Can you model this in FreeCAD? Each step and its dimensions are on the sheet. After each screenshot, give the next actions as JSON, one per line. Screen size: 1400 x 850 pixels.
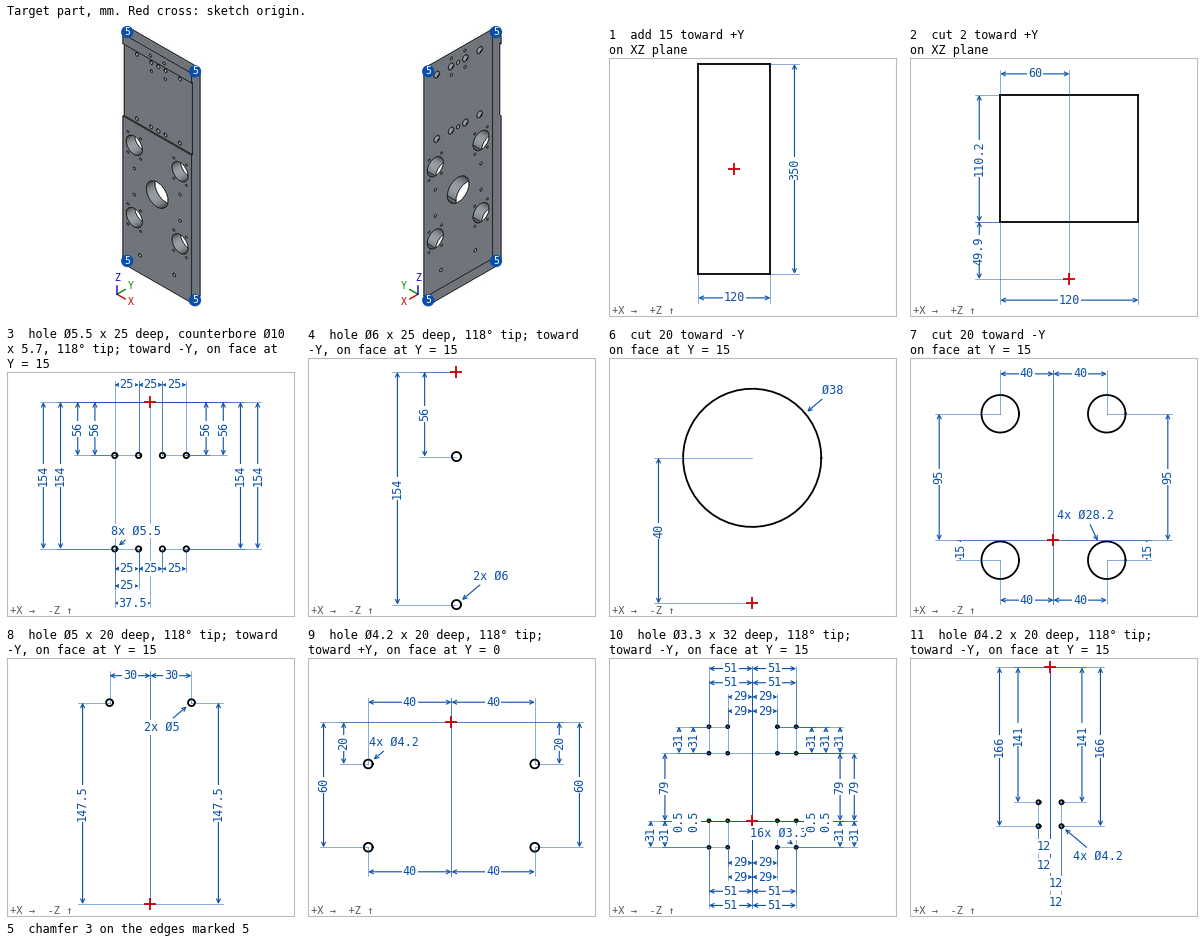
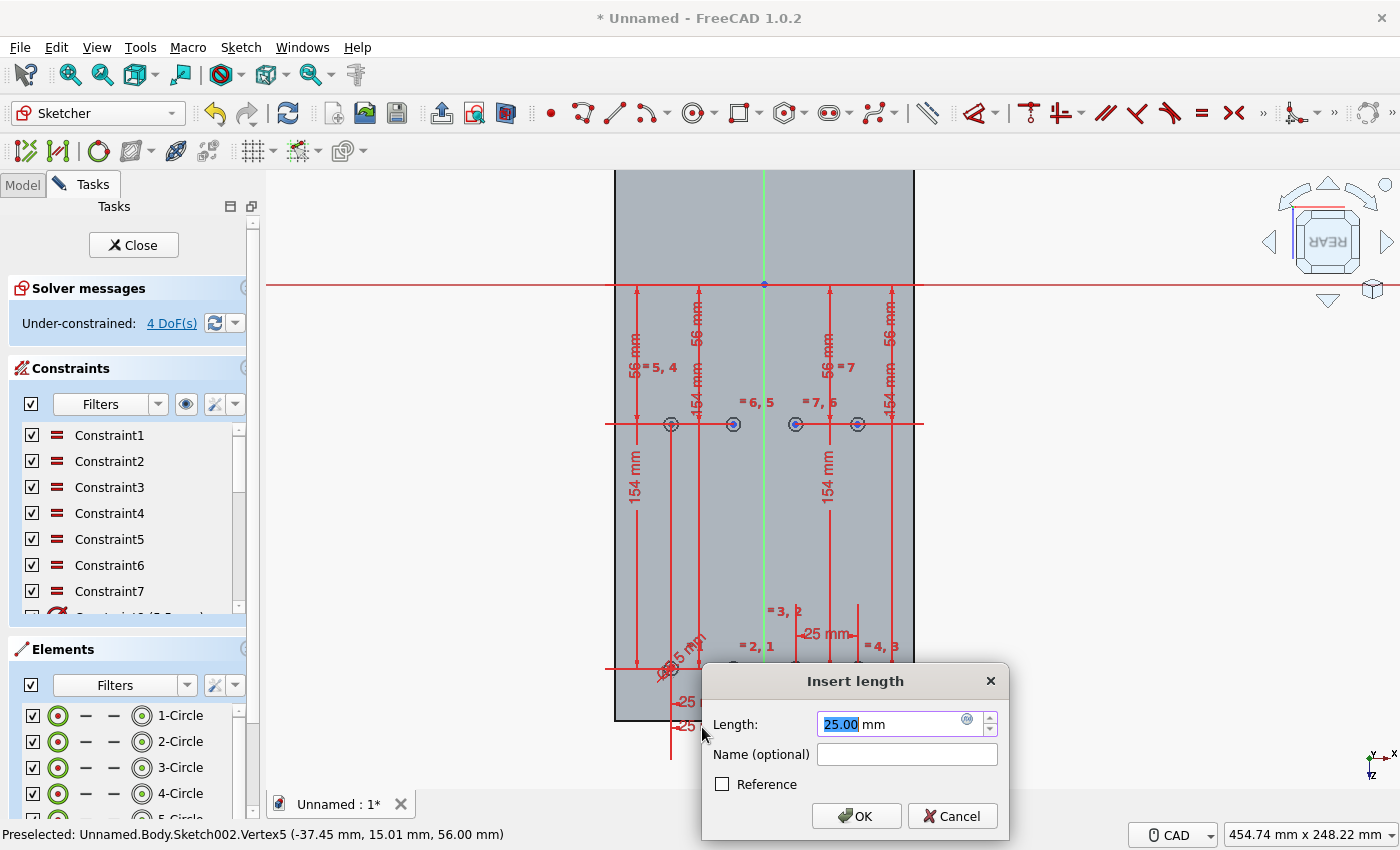
{"action": "type", "text": "25"}
{"action": "key", "text": "Return"}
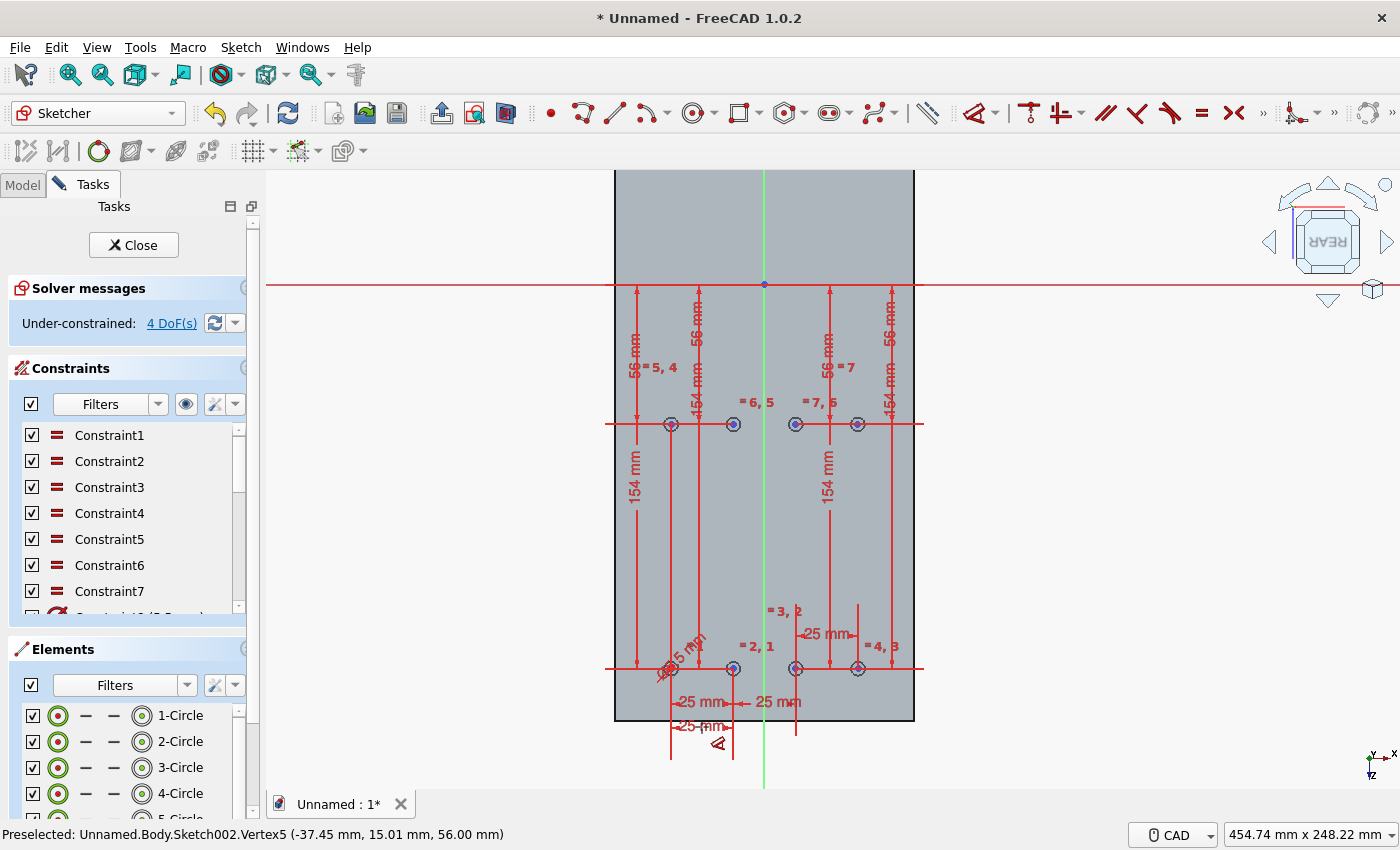
{"action": "left_click", "coordinate": [671, 424]}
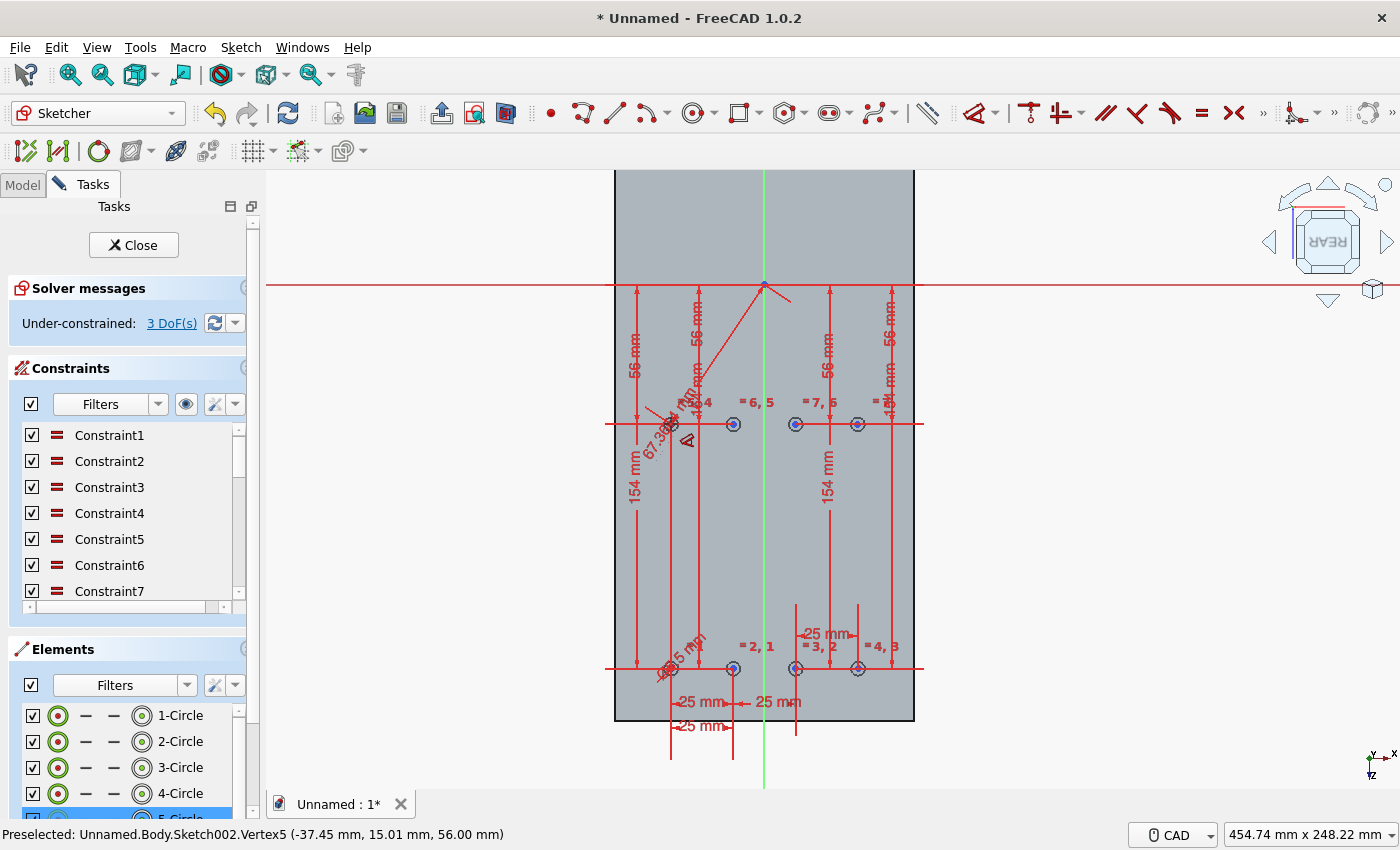
{"action": "left_click", "coordinate": [733, 424]}
{"action": "left_click", "coordinate": [717, 458]}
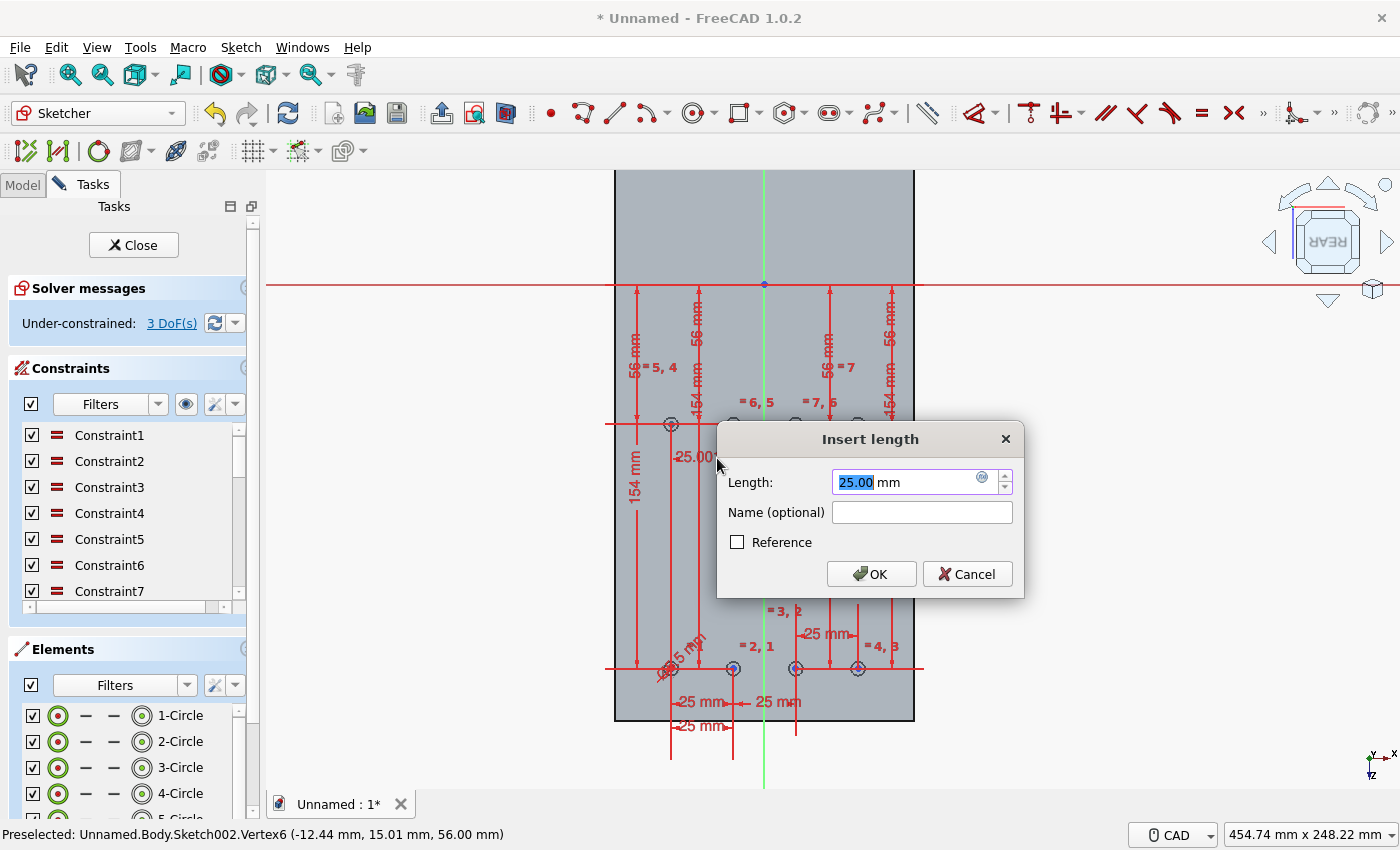
{"action": "type", "text": "25"}
{"action": "key", "text": "Return"}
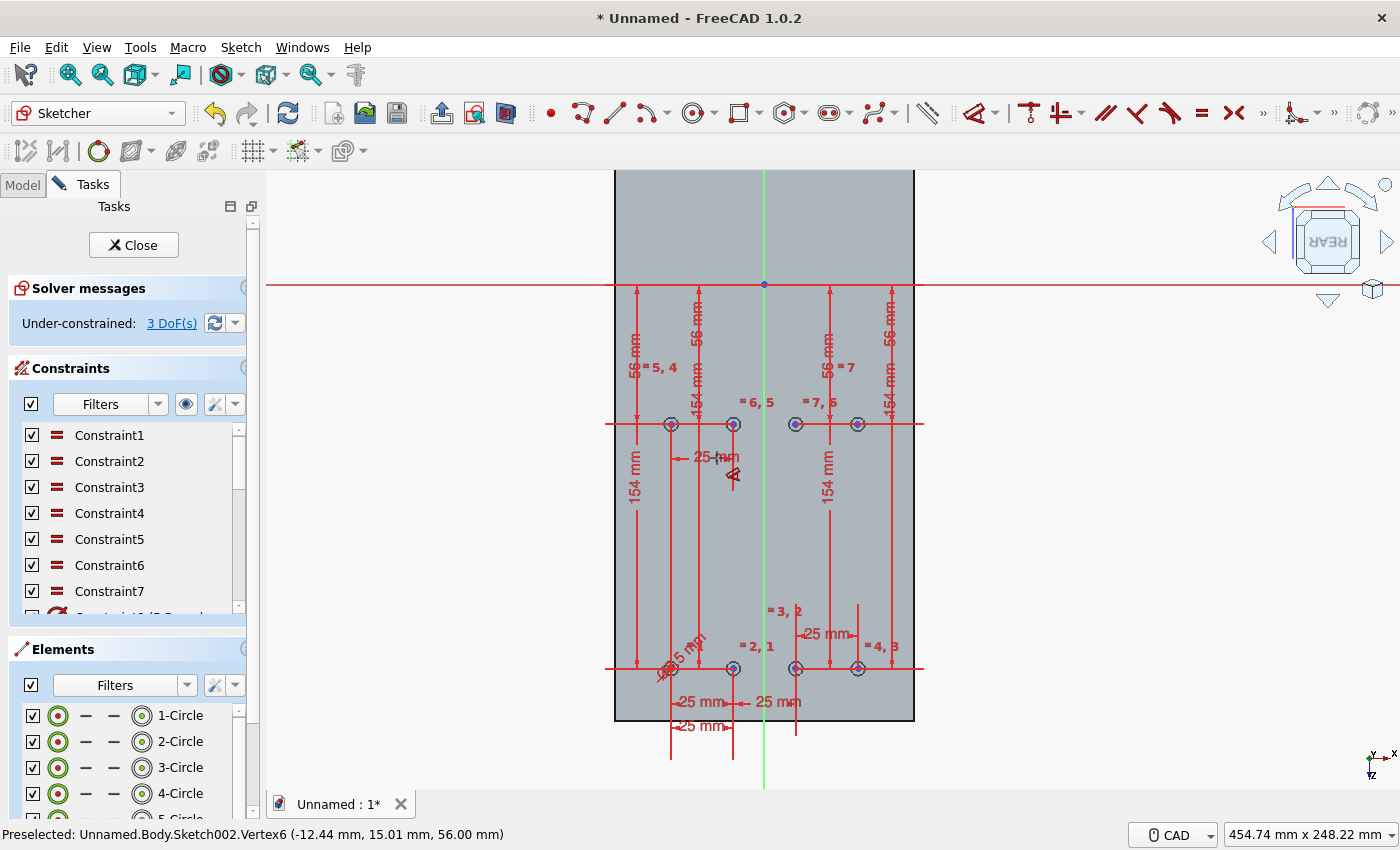
{"action": "left_click", "coordinate": [733, 424]}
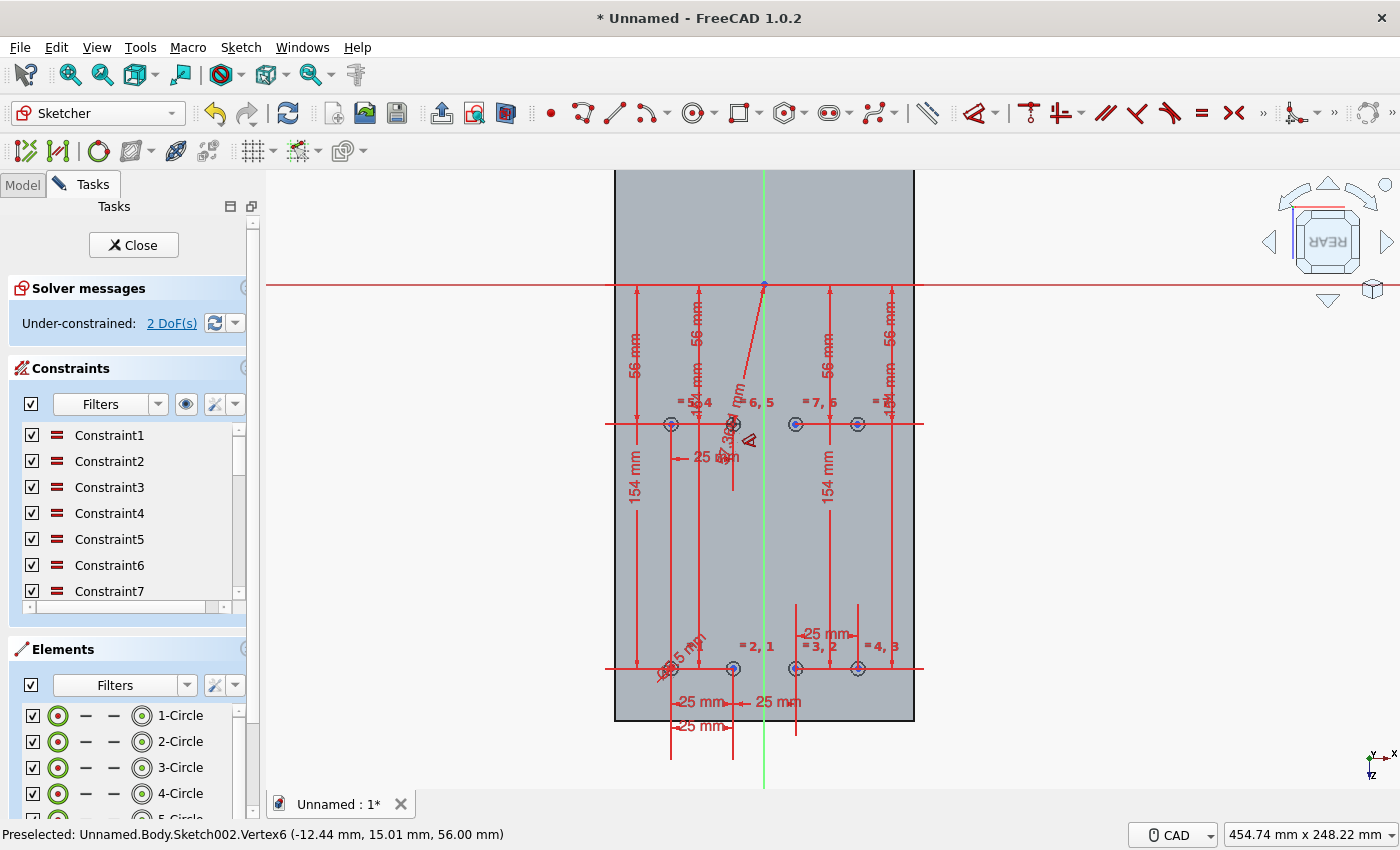
{"action": "left_click", "coordinate": [796, 424]}
{"action": "left_click", "coordinate": [779, 390]}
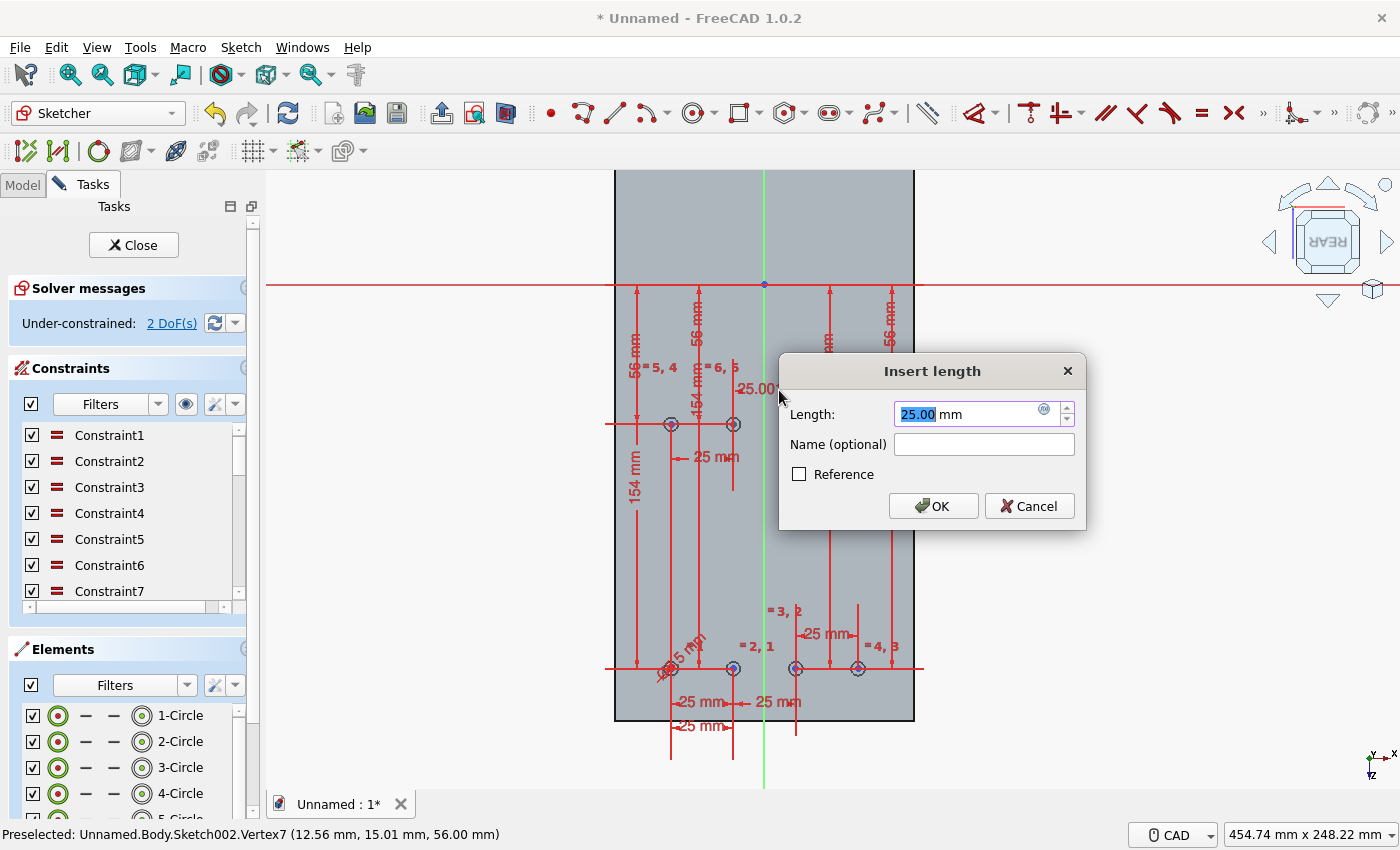
{"action": "type", "text": "25"}
{"action": "key", "text": "Return"}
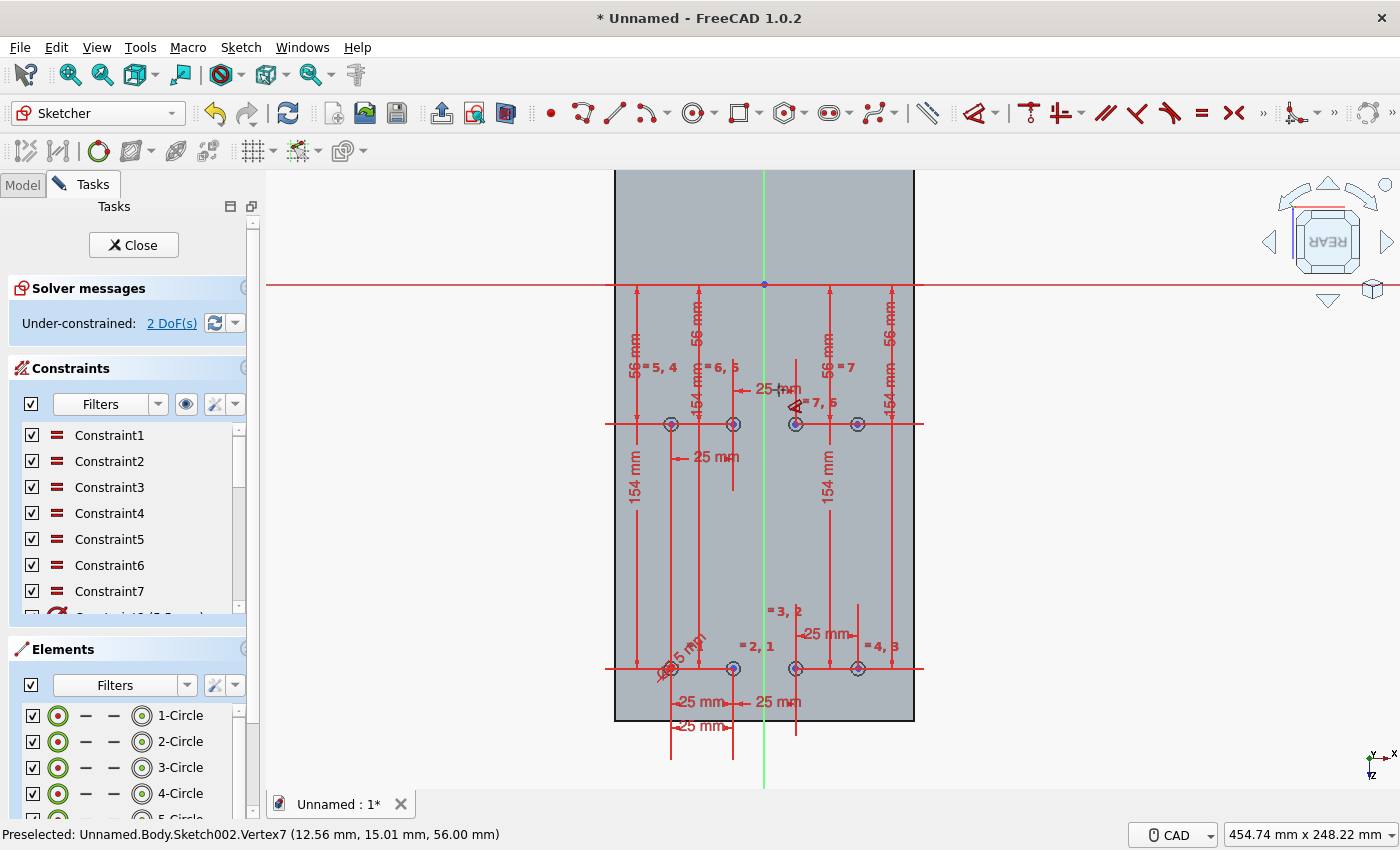
{"action": "left_click", "coordinate": [796, 424]}